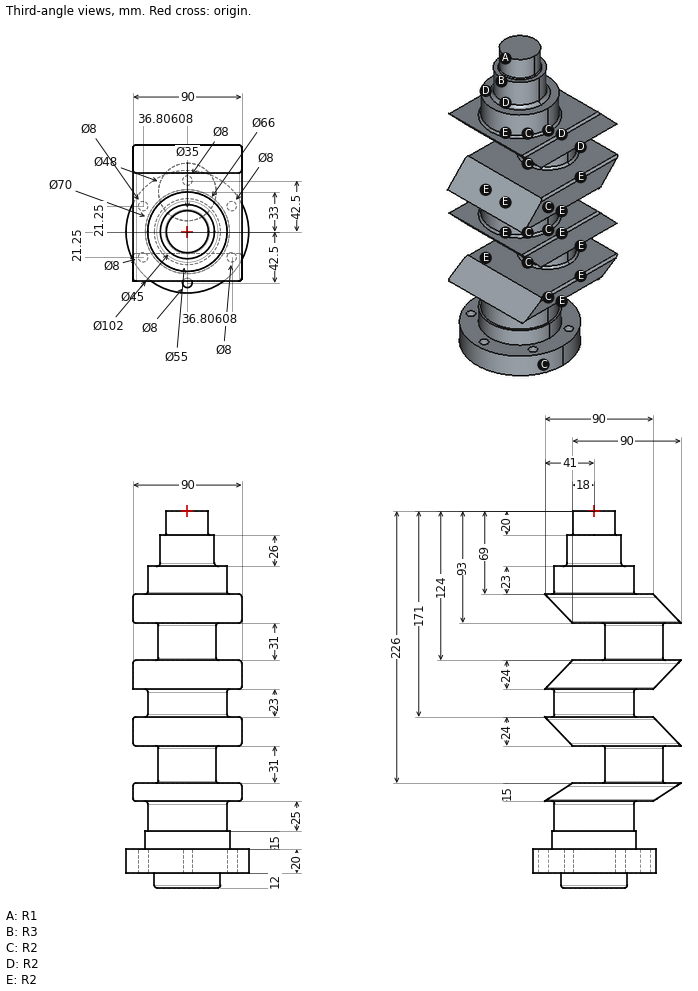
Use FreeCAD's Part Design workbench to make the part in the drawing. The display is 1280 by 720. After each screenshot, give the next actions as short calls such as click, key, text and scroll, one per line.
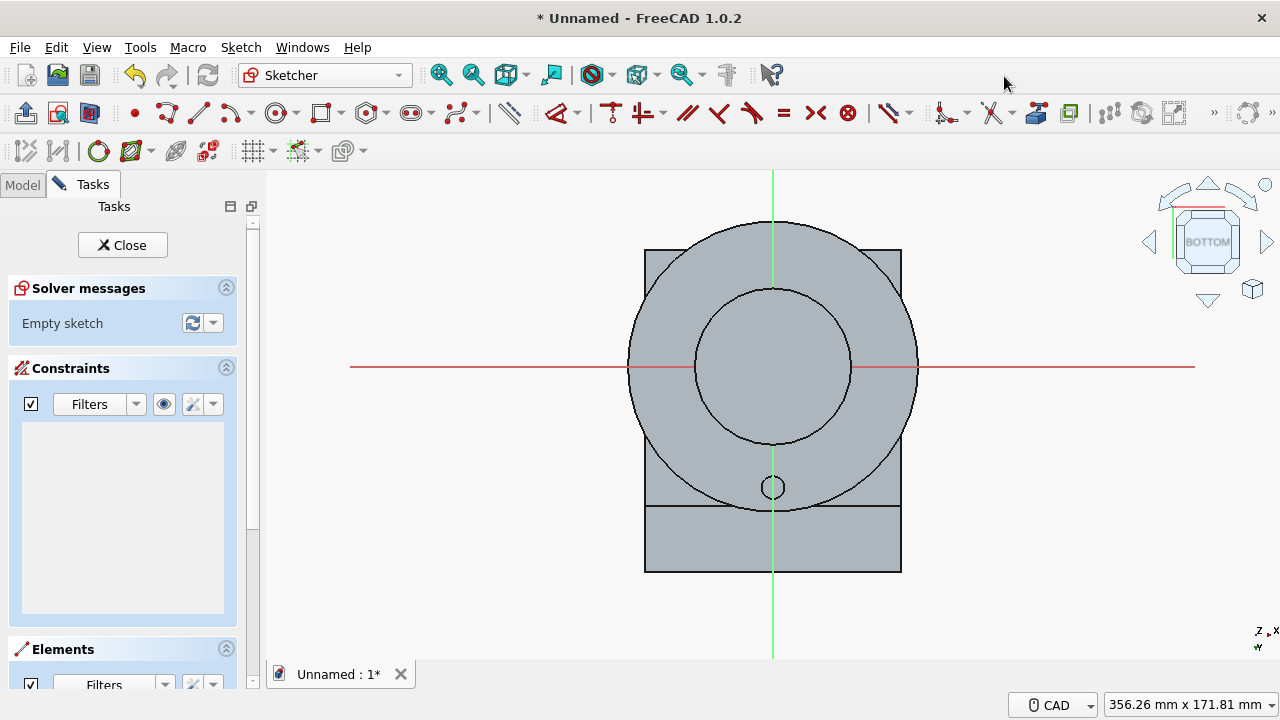
click(90, 114)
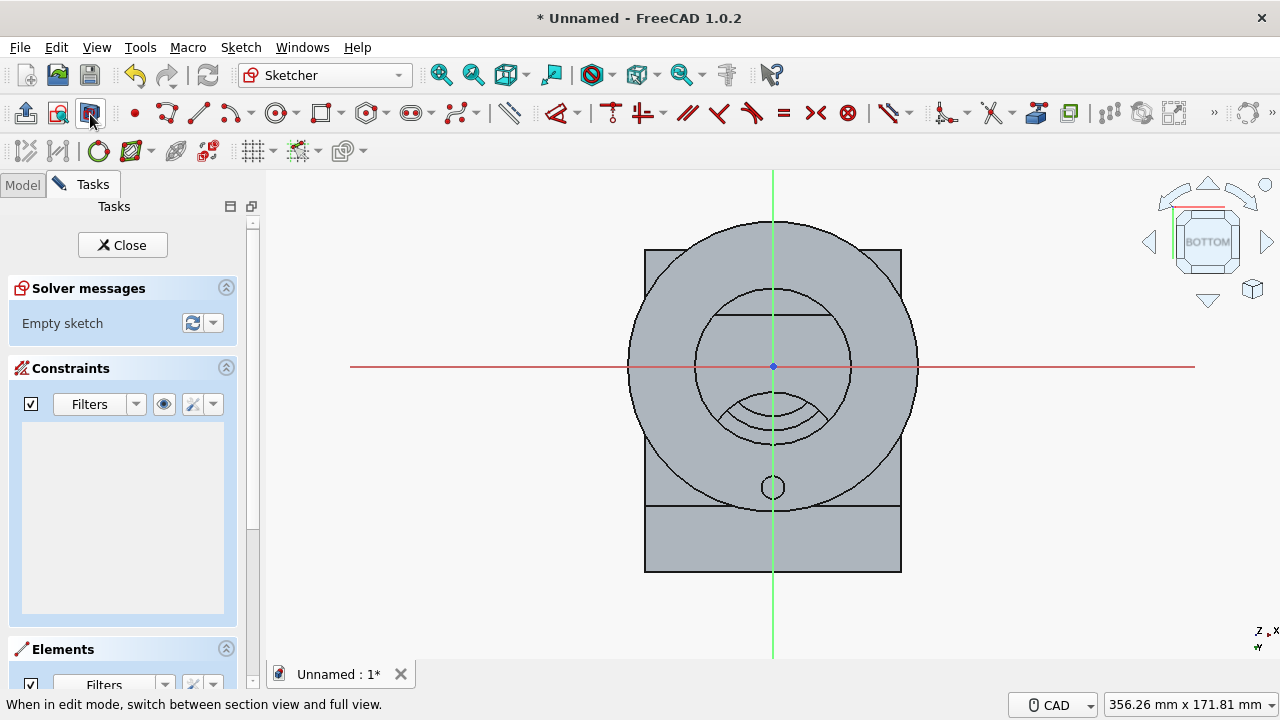
scroll(665, 428, up, 13)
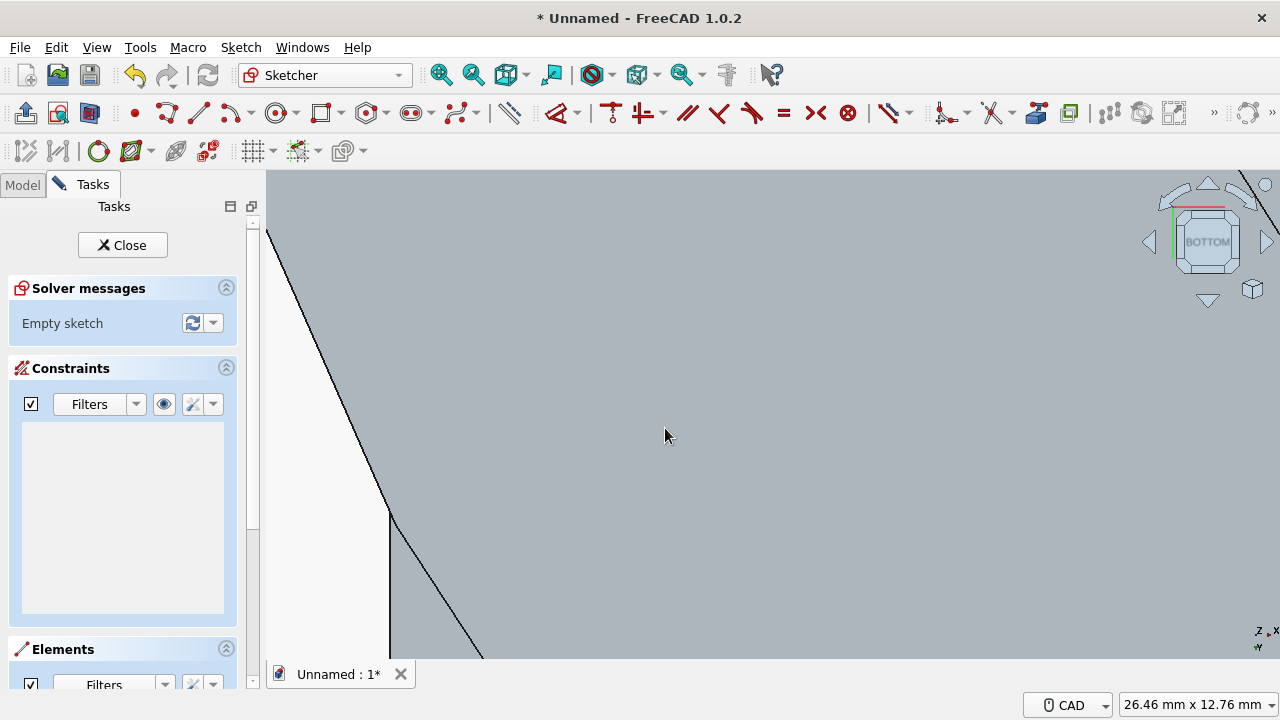
click(276, 114)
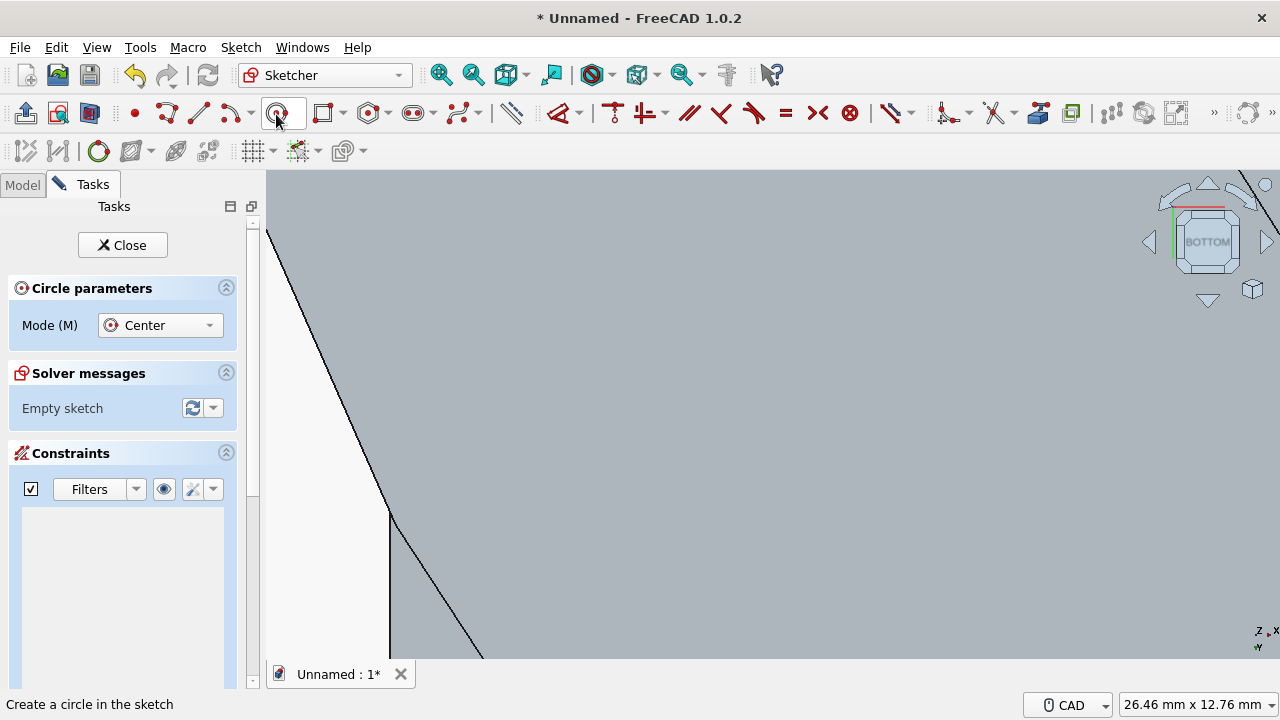
click(704, 409)
move(813, 301)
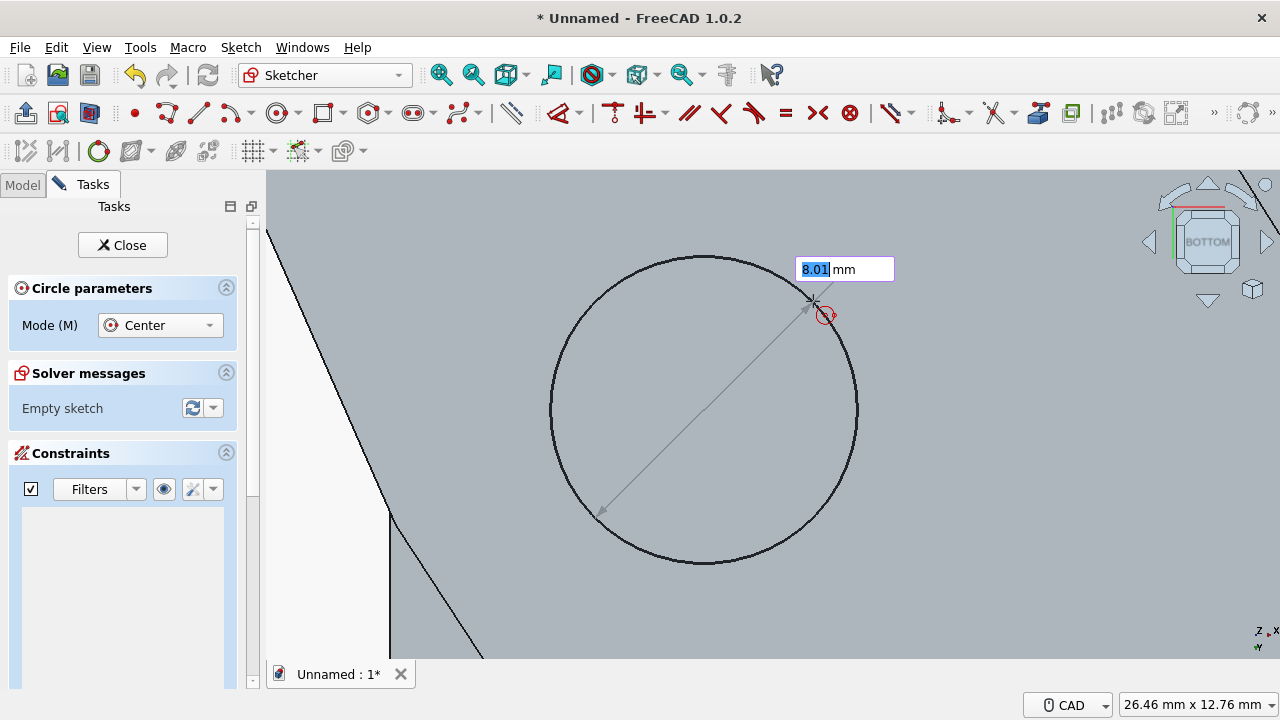
text(8)
key(Return)
key(Escape)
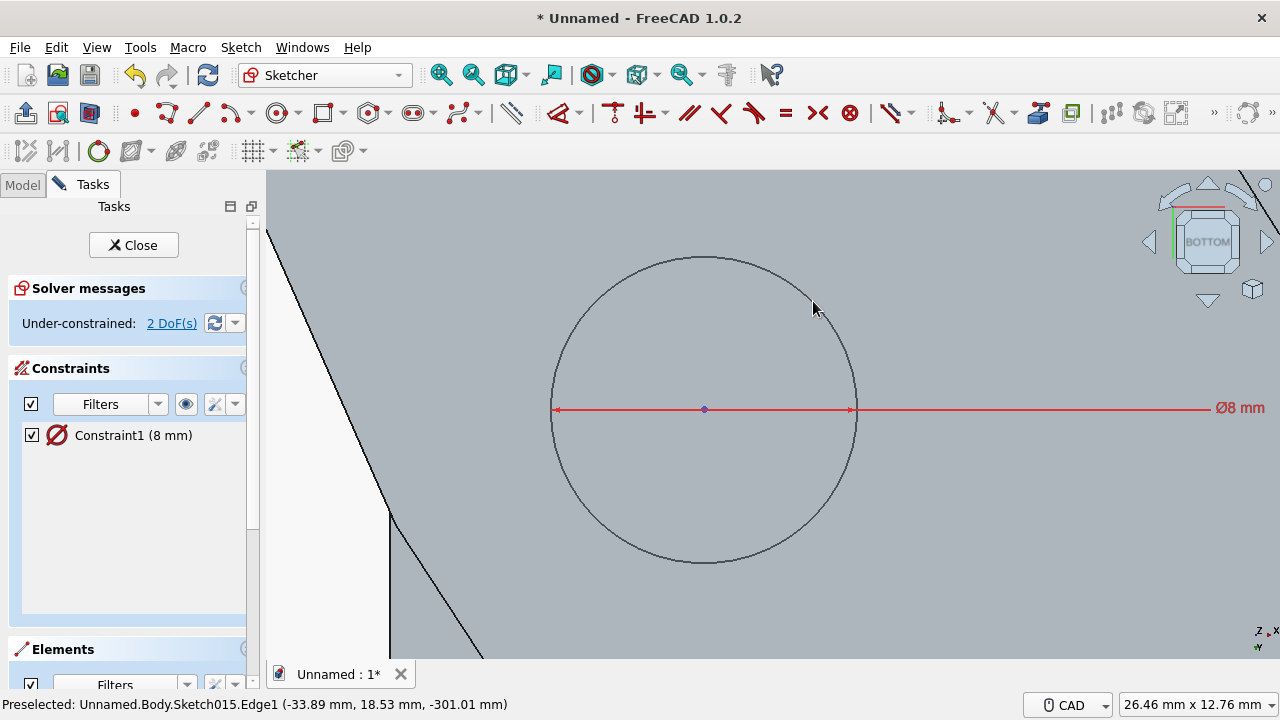
click(558, 114)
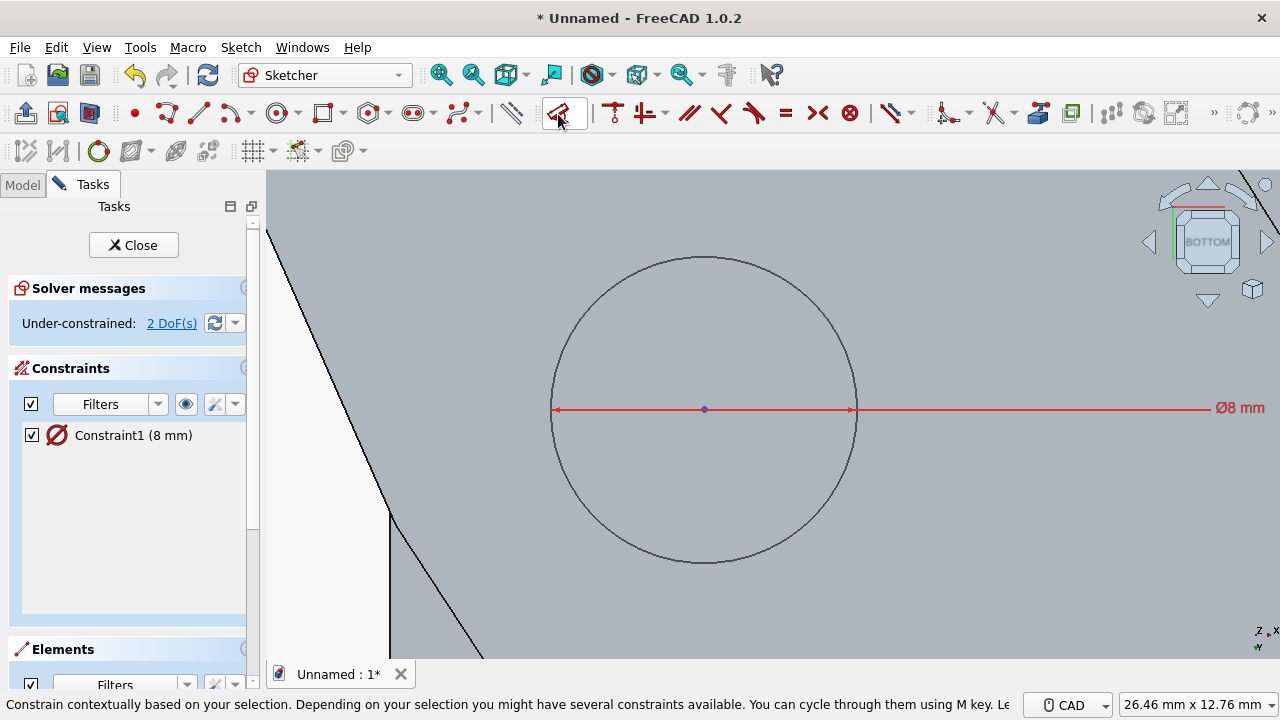
click(704, 410)
click(670, 304)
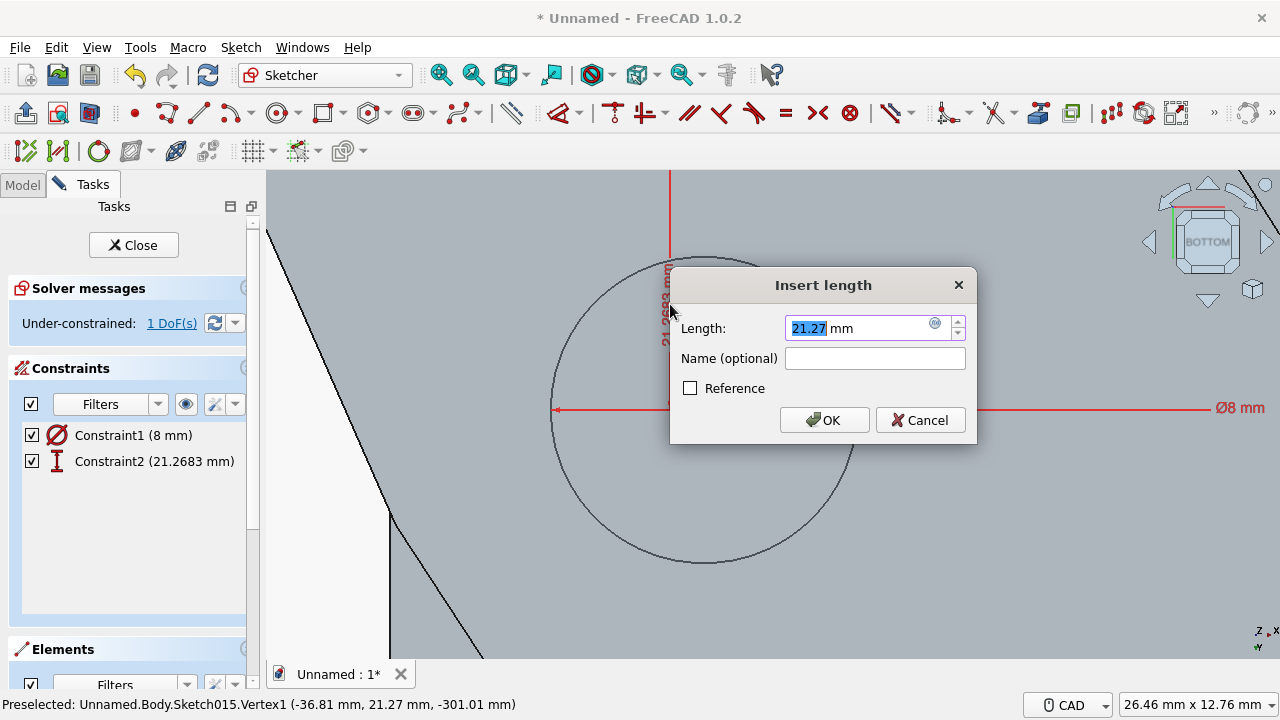
text(21.25)
key(Return)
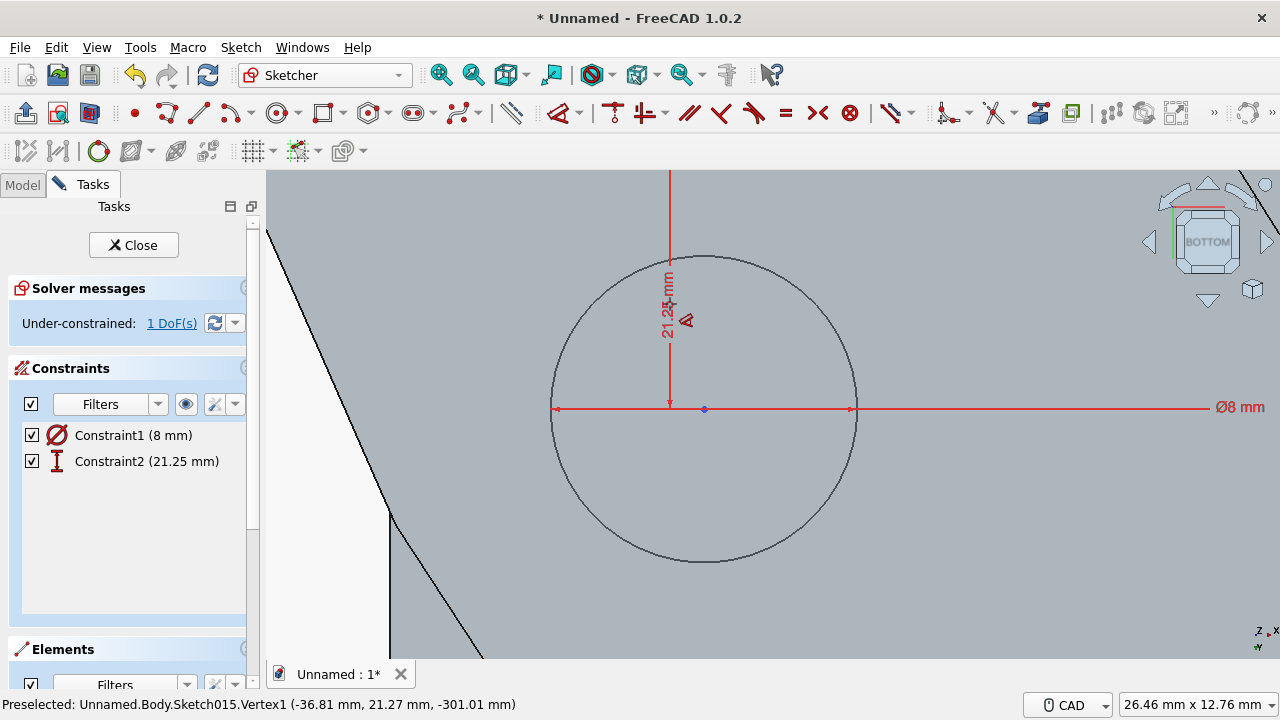
click(704, 409)
click(909, 443)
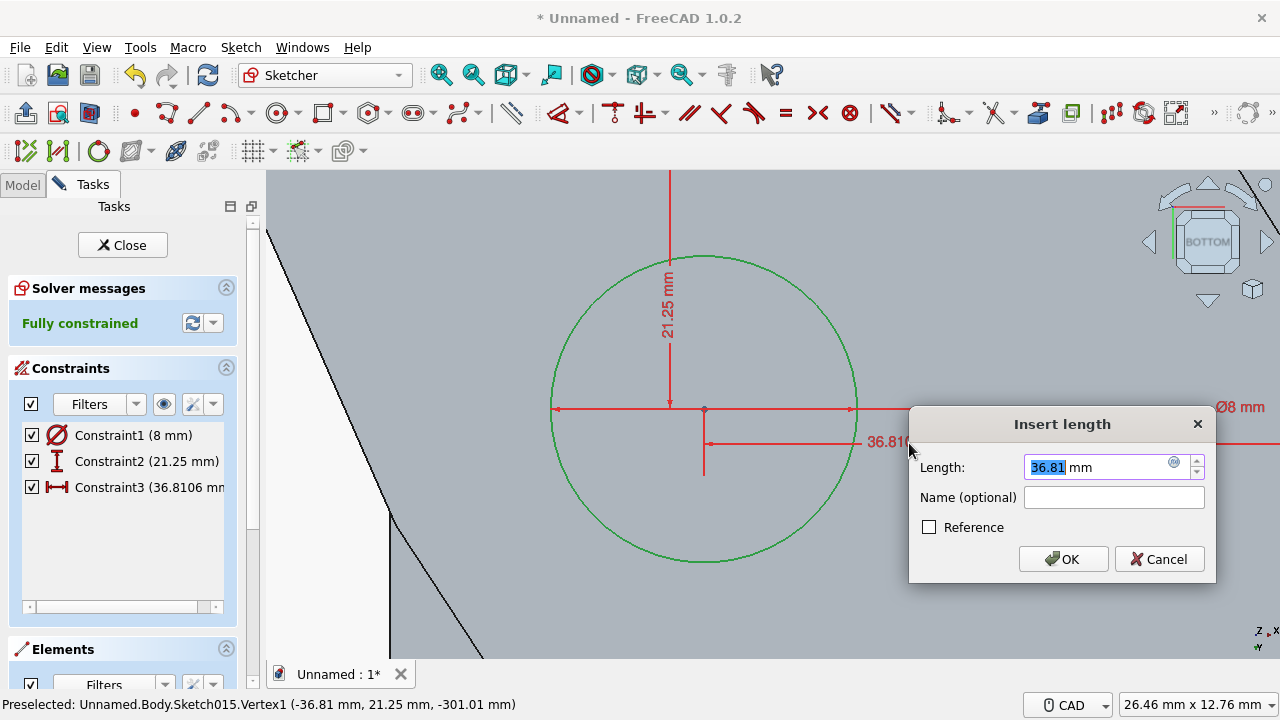
text(36.80608)
key(Return)
key(Escape)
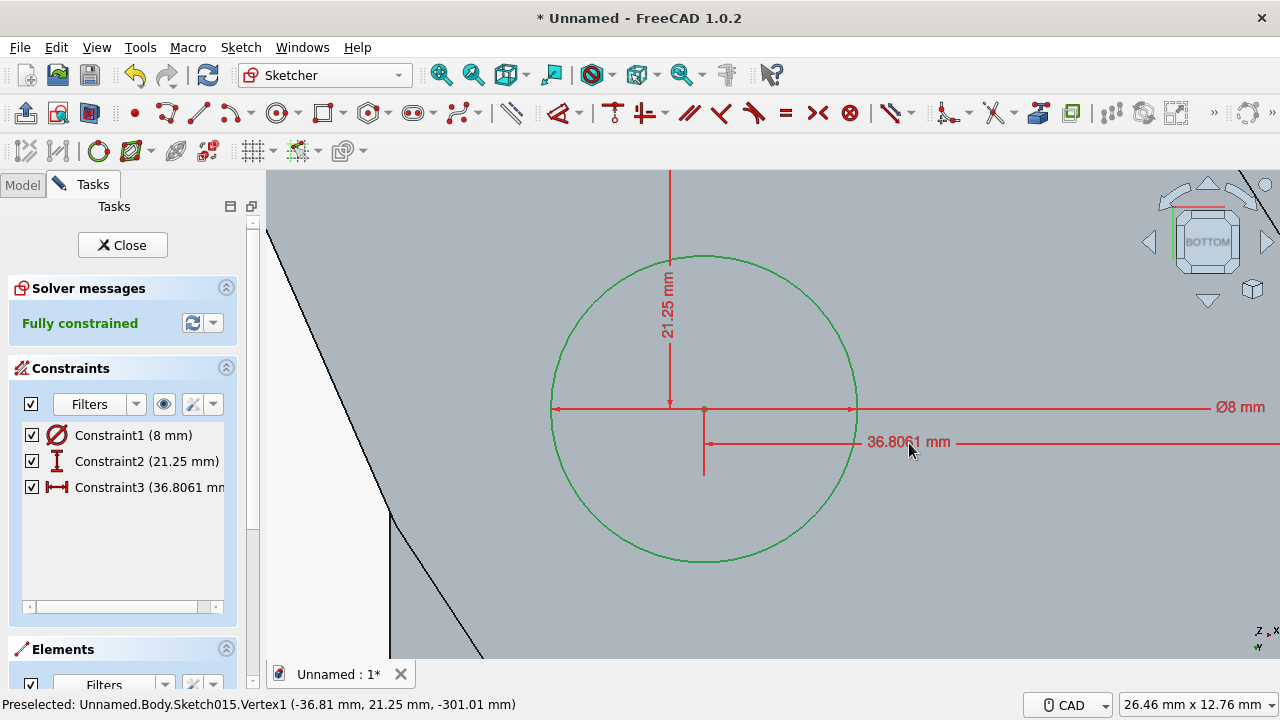
click(123, 245)